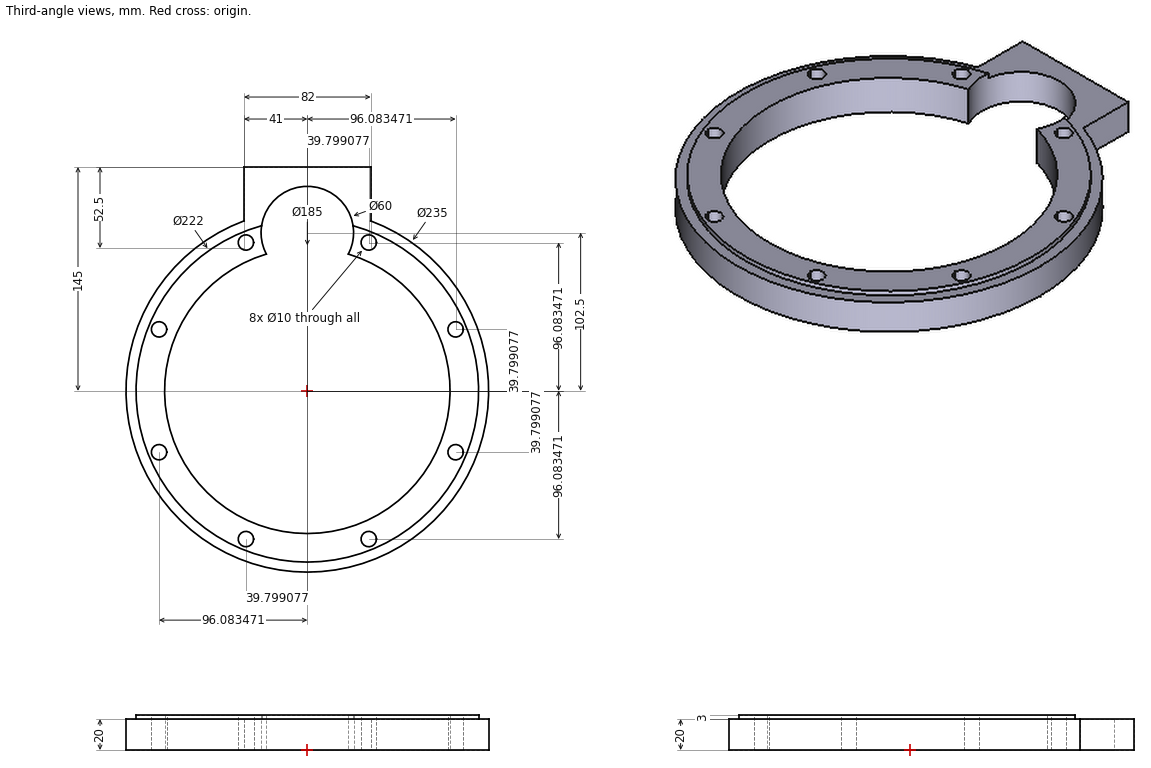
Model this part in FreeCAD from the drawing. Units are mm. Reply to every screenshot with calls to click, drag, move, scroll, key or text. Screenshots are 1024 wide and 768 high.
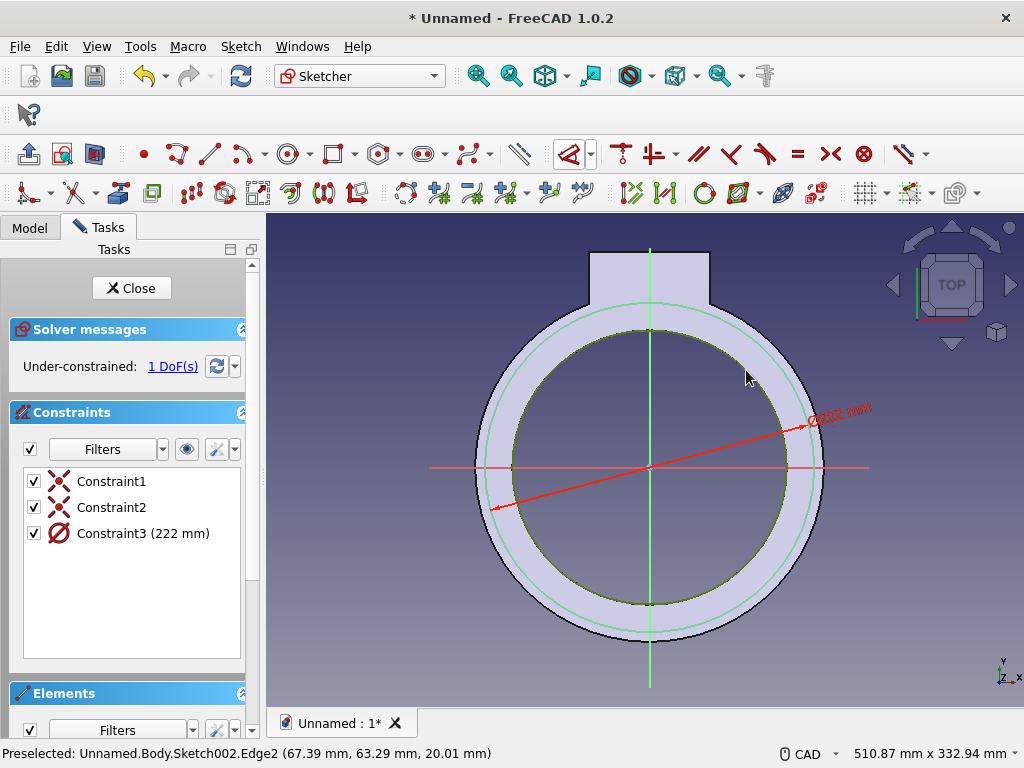
key(k)
key(o)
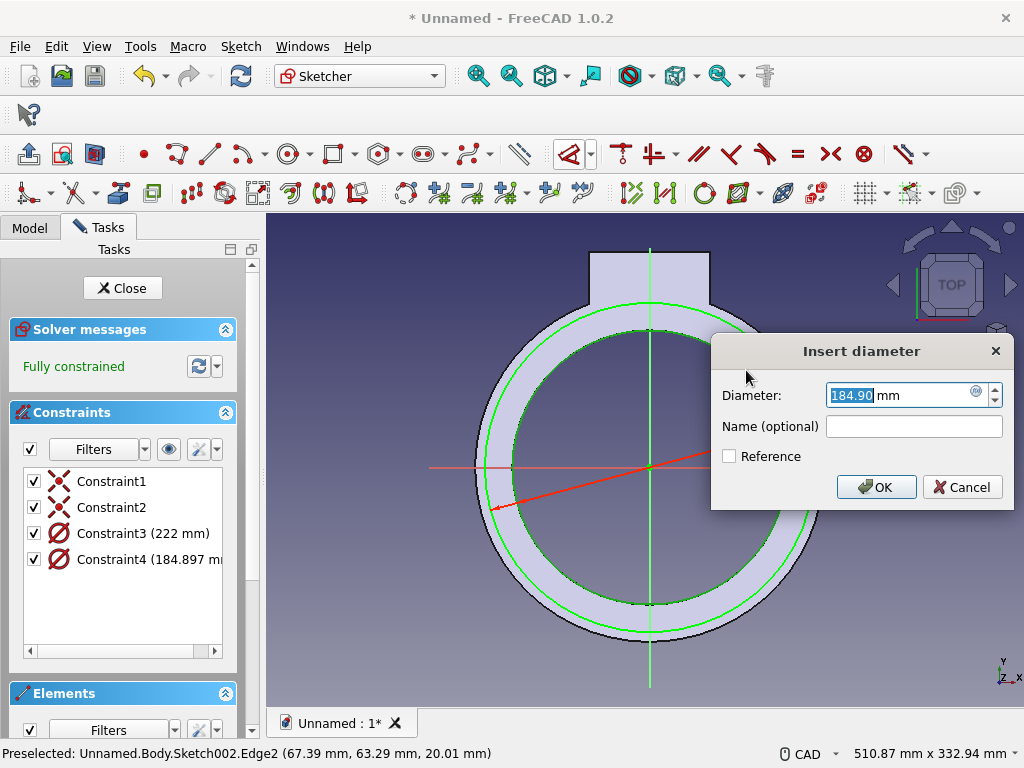
text(185)
key(Return)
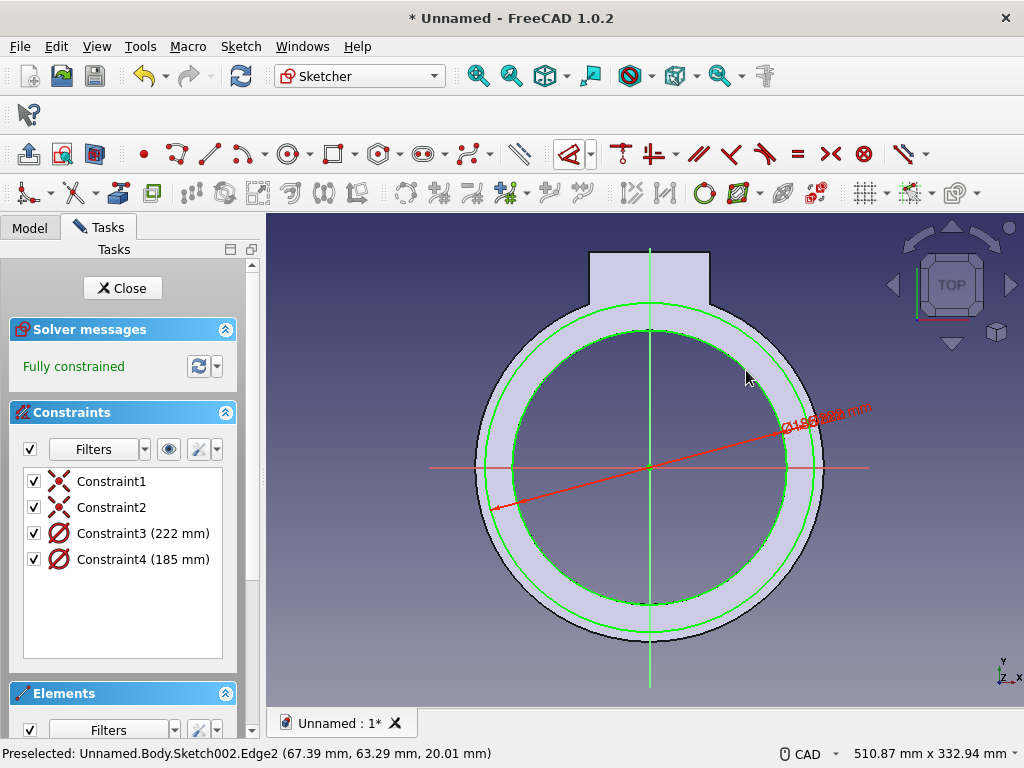
click(123, 288)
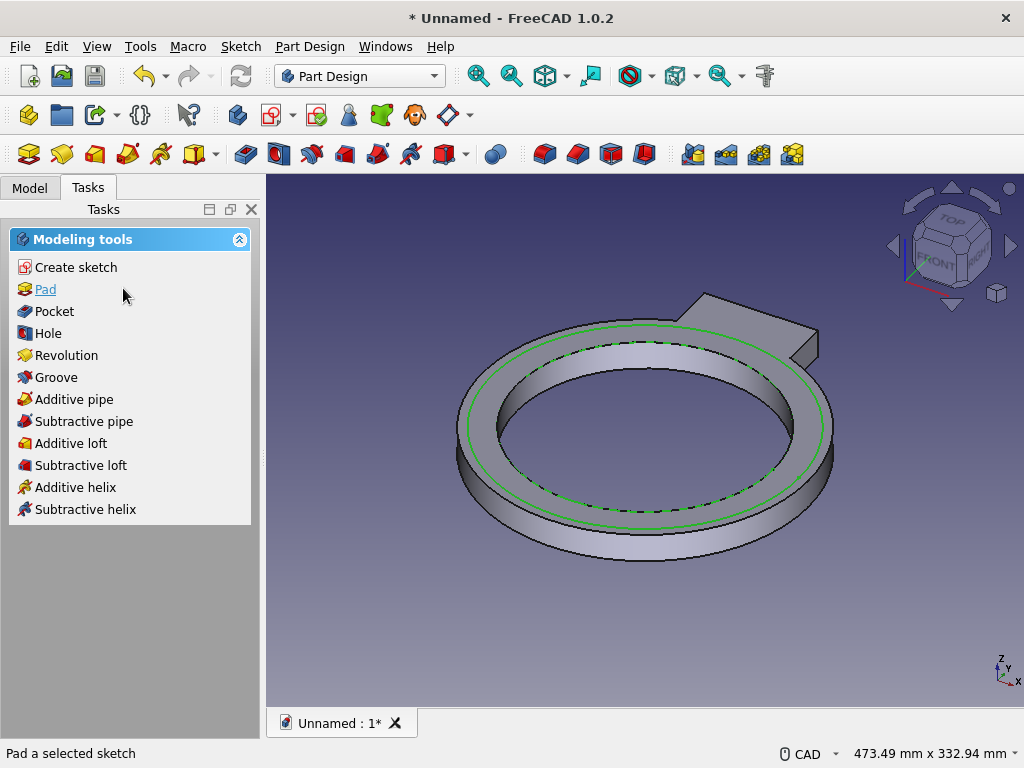
click(29, 154)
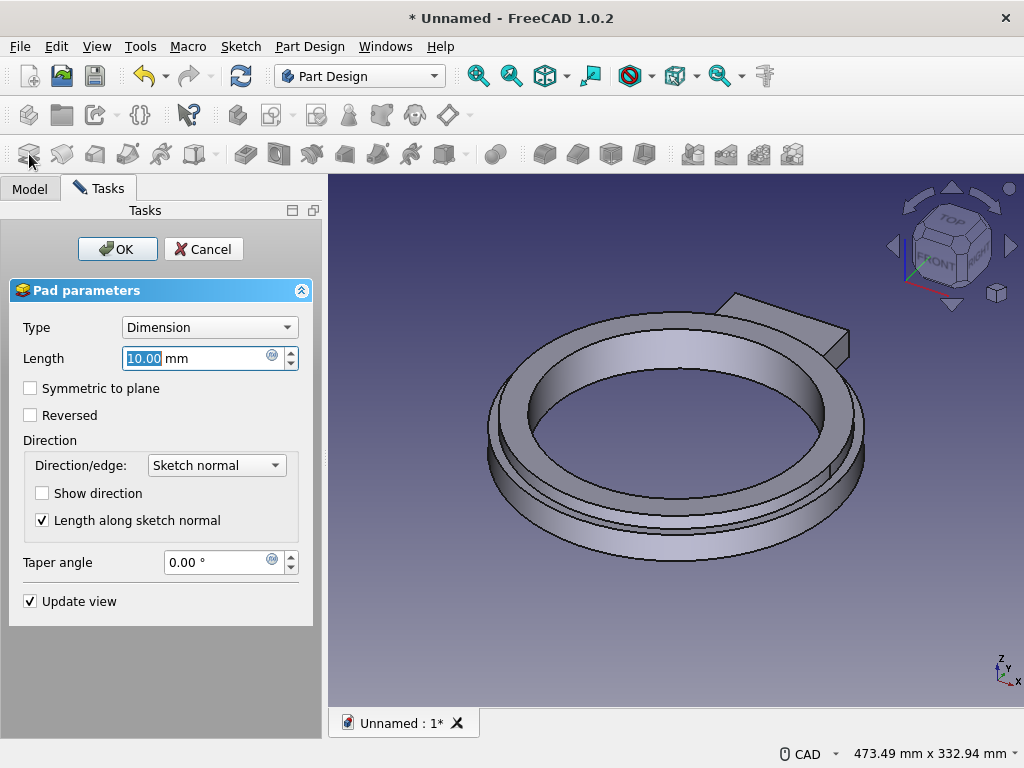
text(3)
key(Tab)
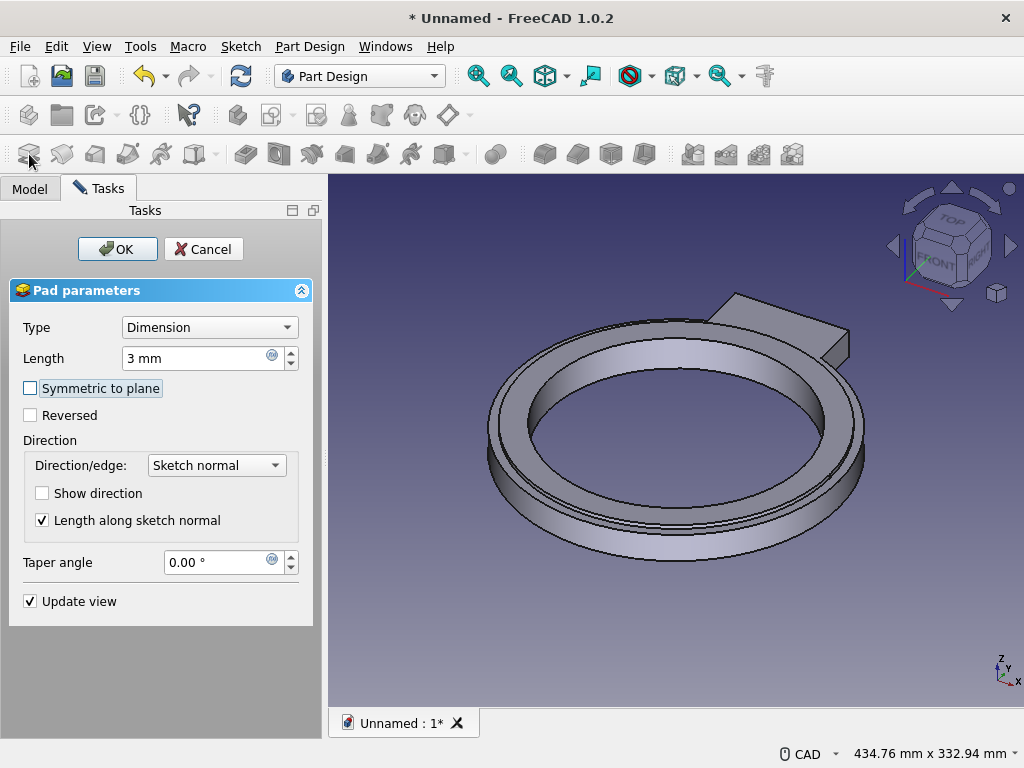
click(118, 249)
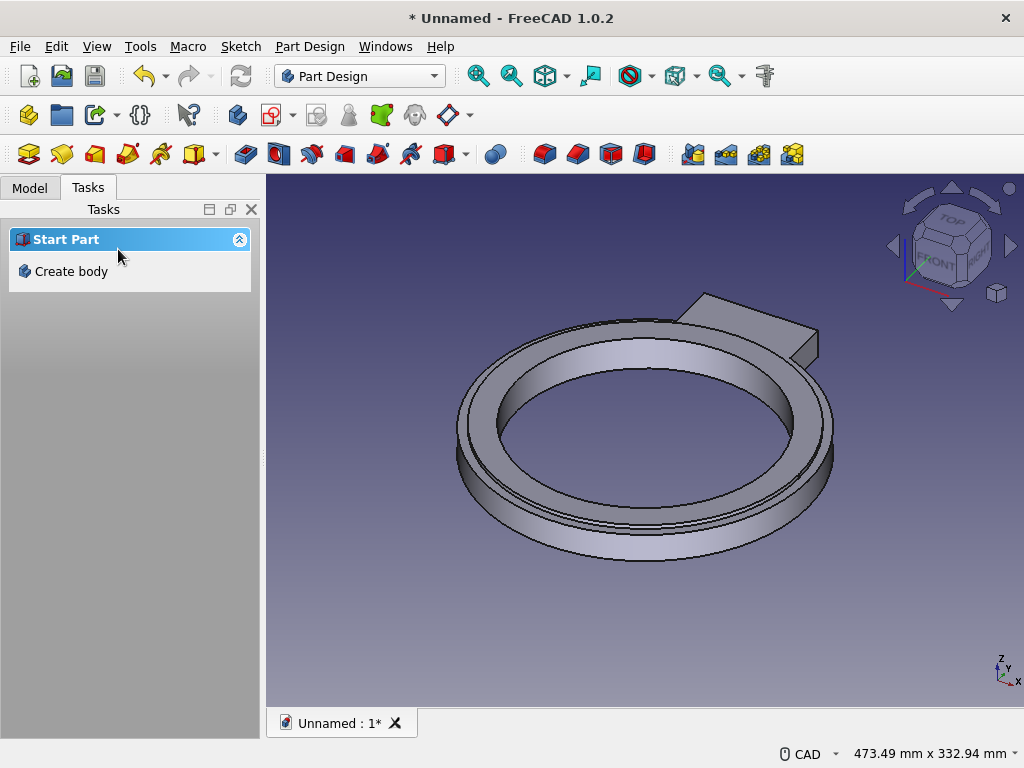
key(5)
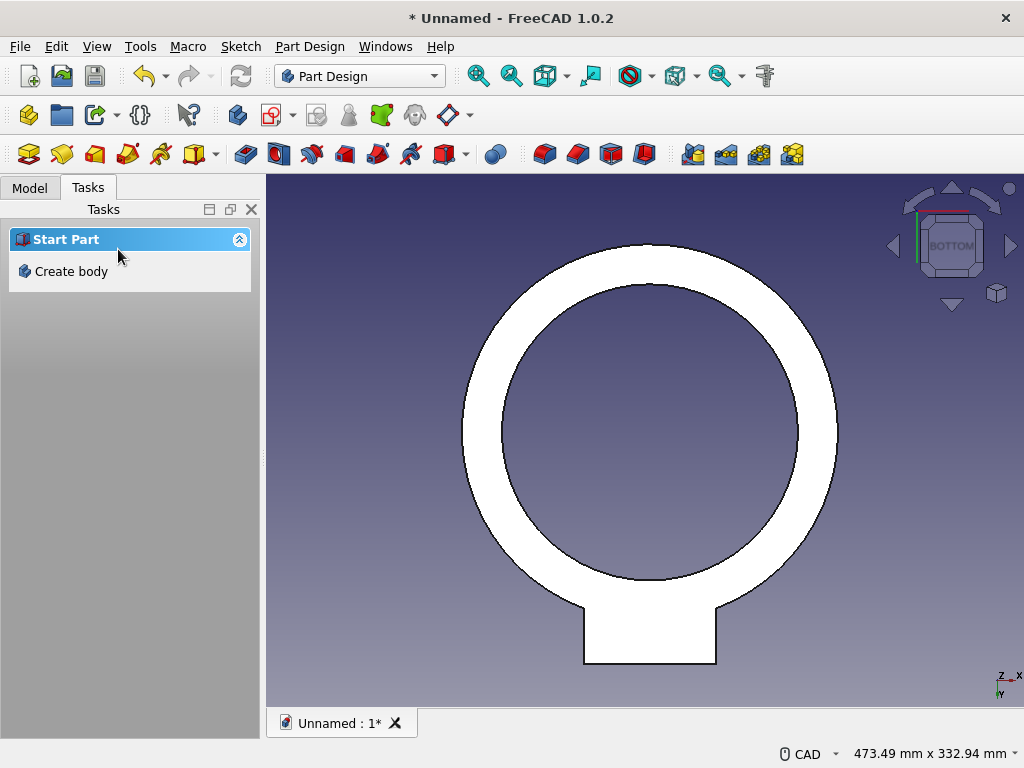
click(650, 633)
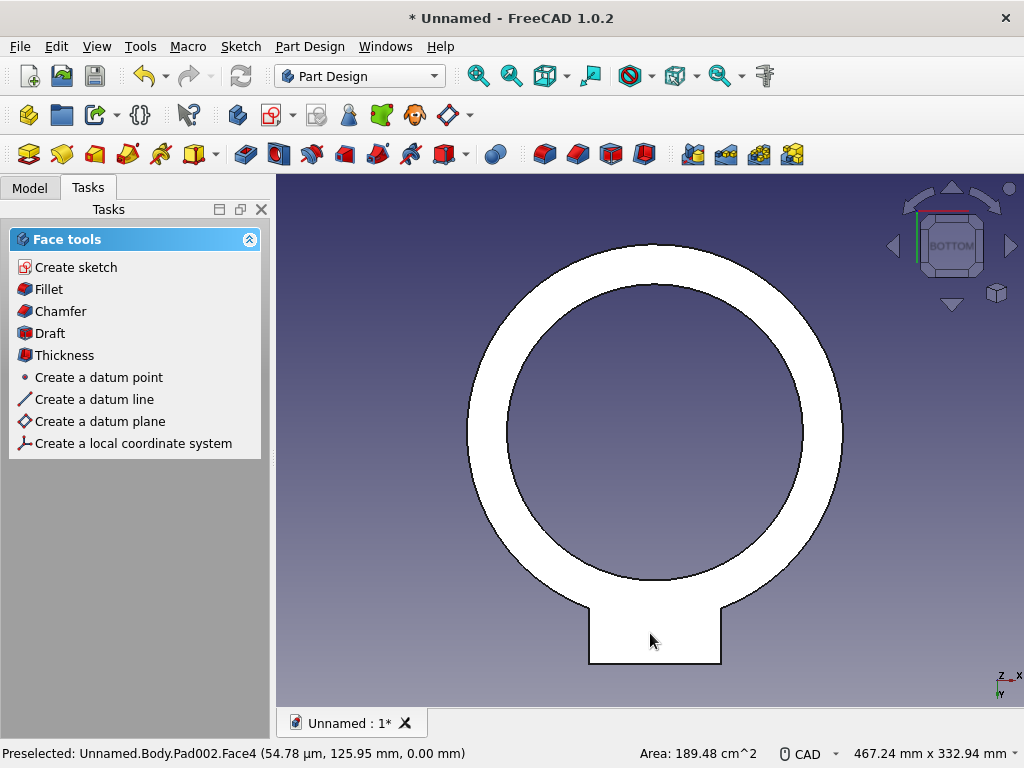
click(270, 116)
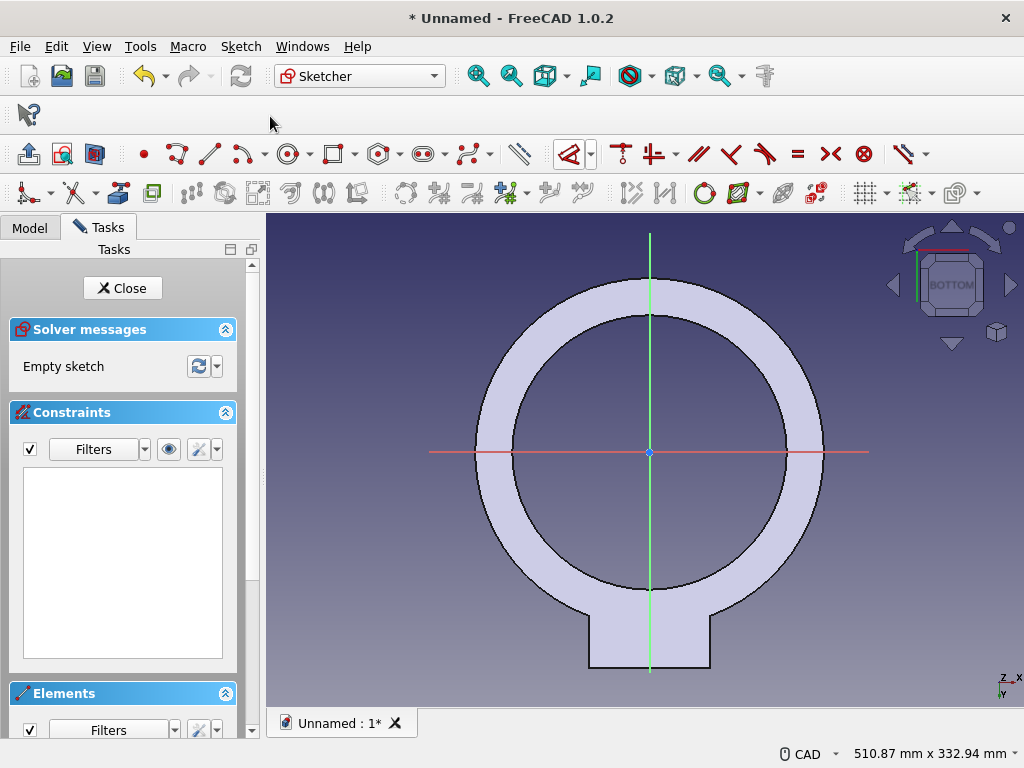
scroll(798, 679, up, 2)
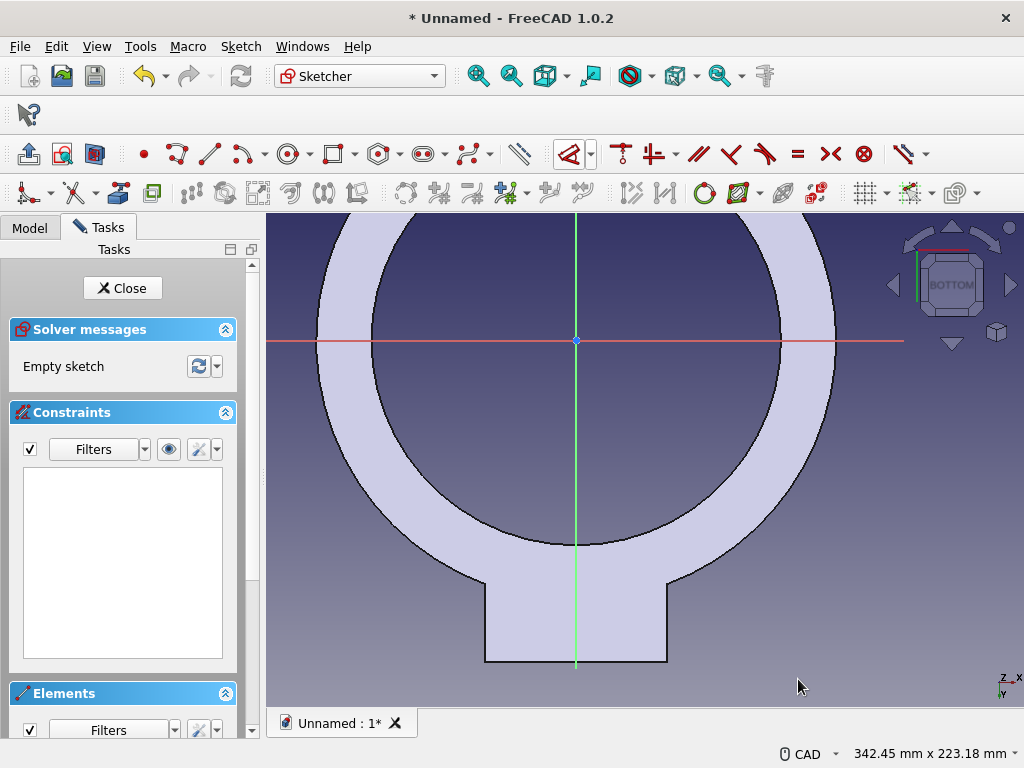
click(288, 154)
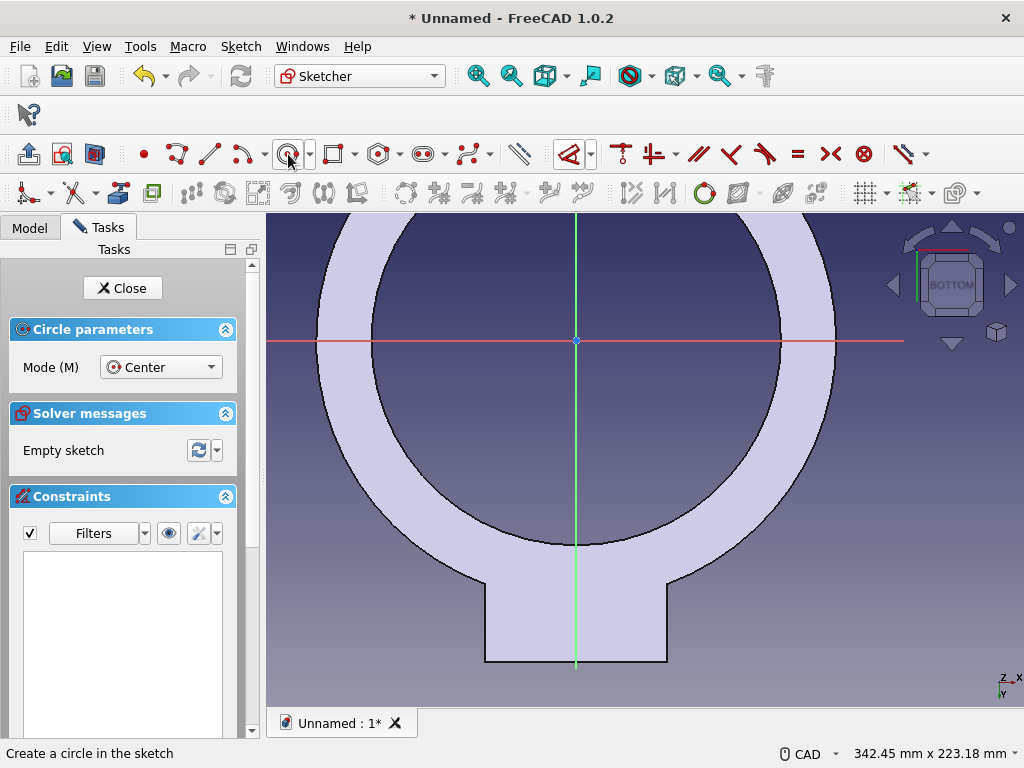
click(576, 567)
click(623, 521)
key(Escape)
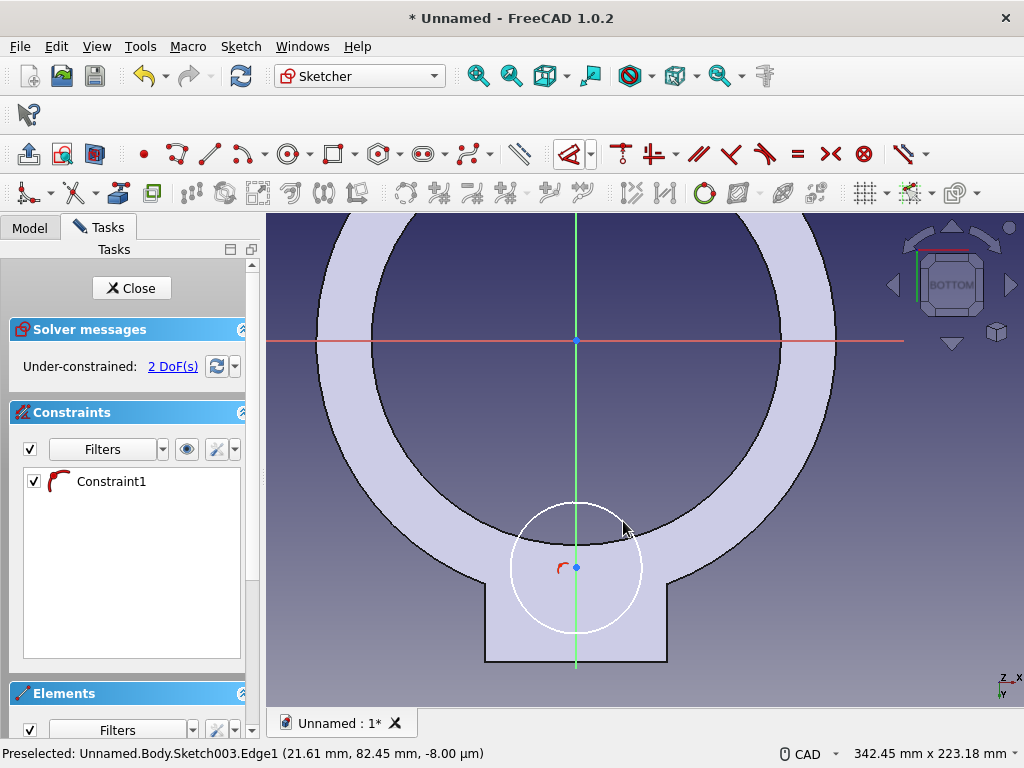
click(622, 521)